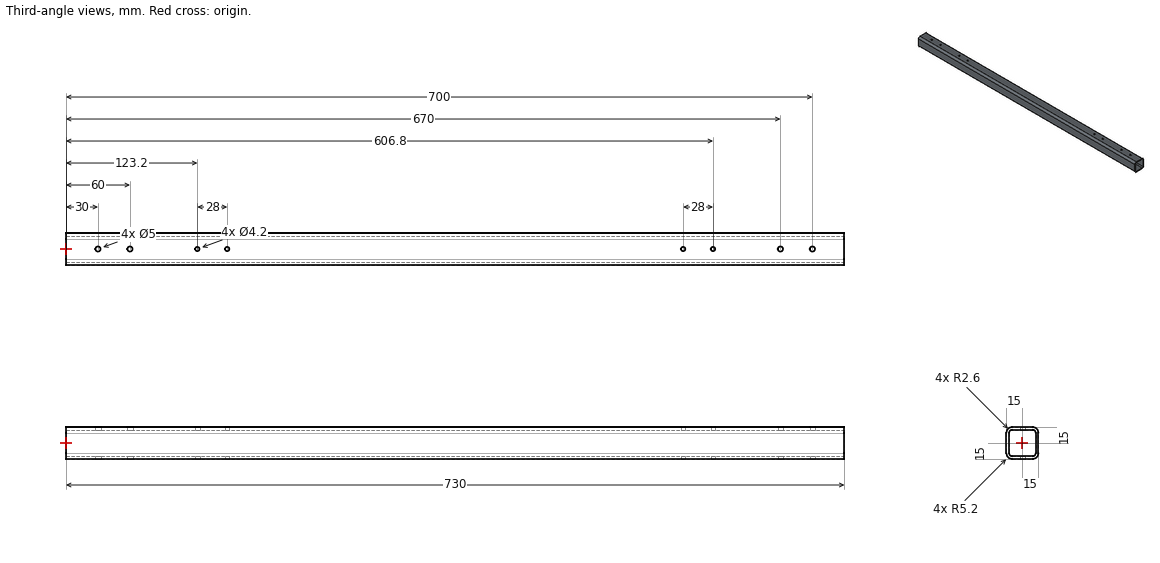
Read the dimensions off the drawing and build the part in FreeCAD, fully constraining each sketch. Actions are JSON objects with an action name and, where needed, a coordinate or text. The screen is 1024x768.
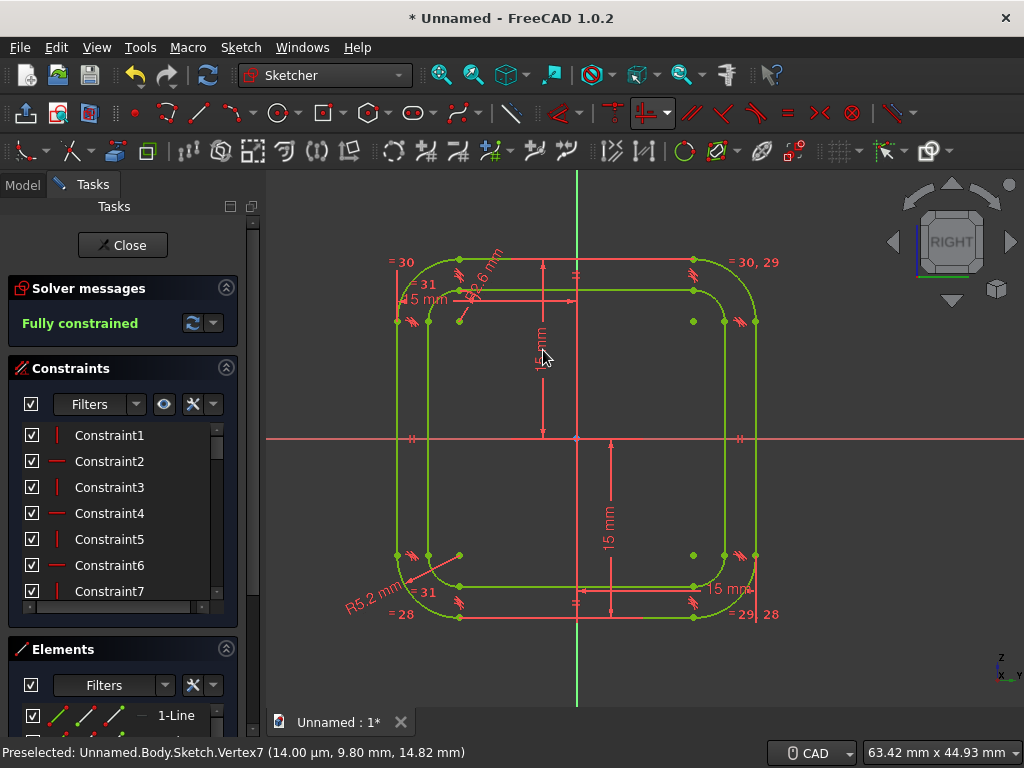
{"action": "left_click", "coordinate": [123, 245]}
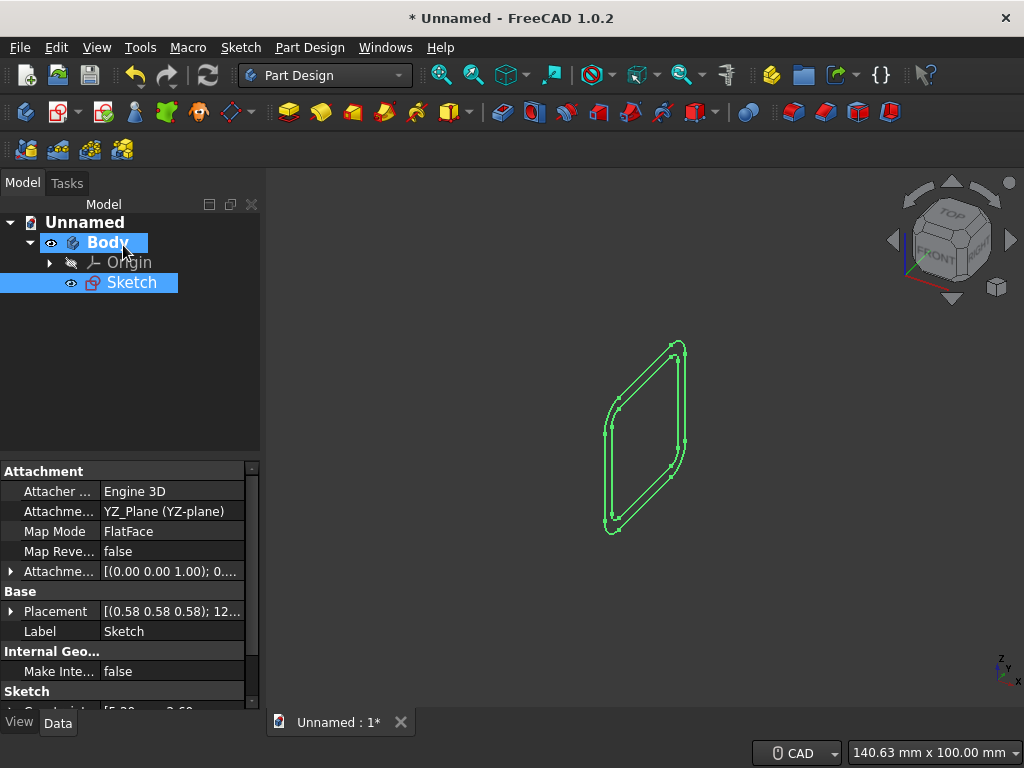
{"action": "left_click", "coordinate": [290, 112]}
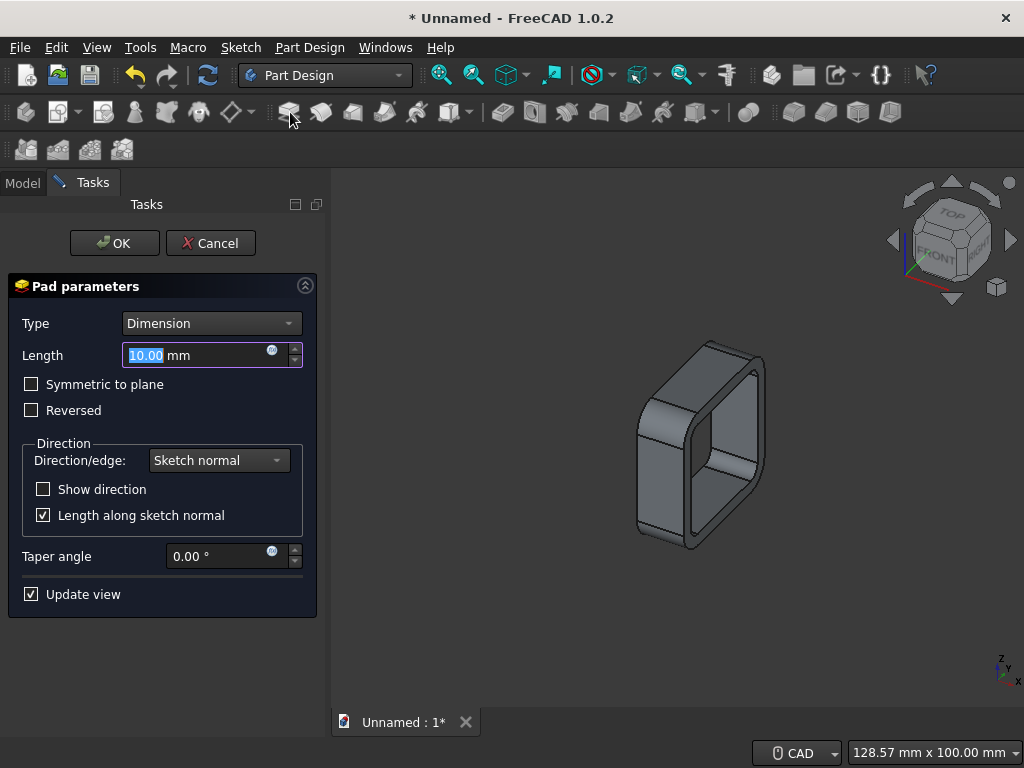
{"action": "type", "text": "730"}
{"action": "key", "text": "Tab"}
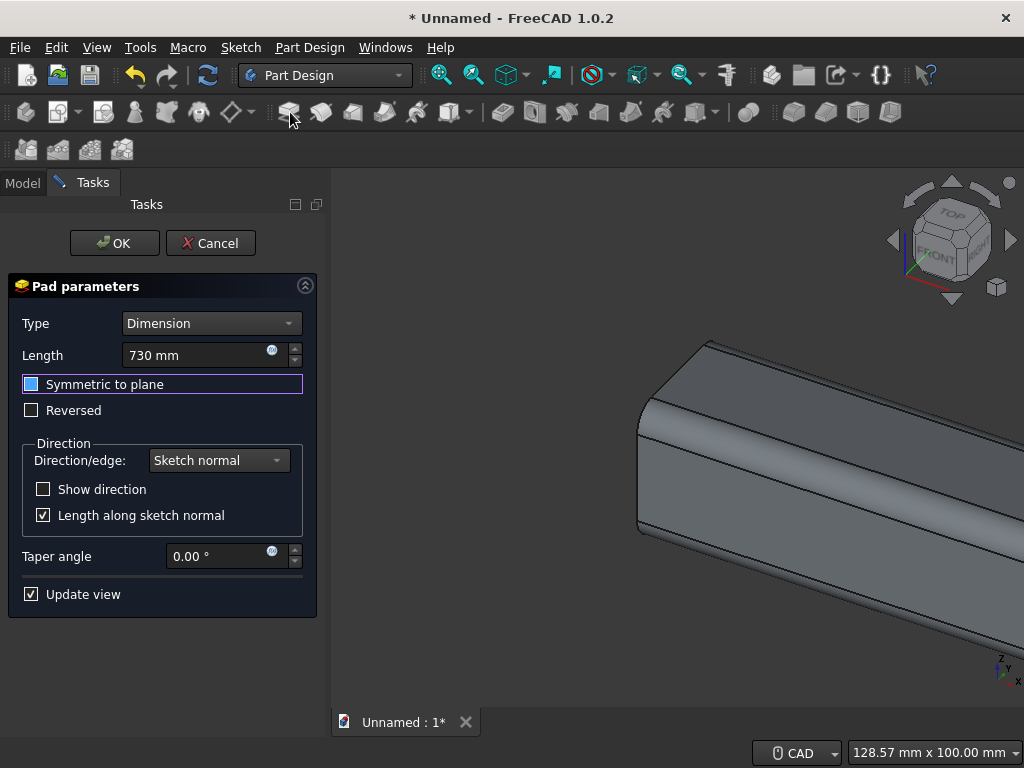
{"action": "left_click", "coordinate": [115, 243]}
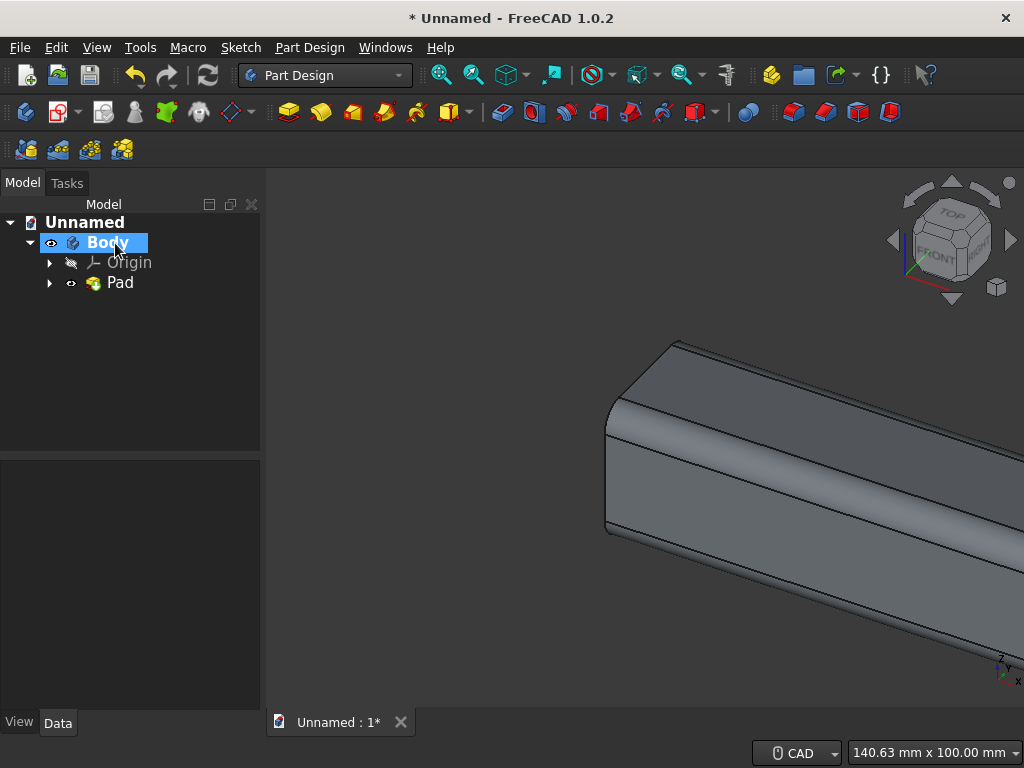
{"action": "left_click", "coordinate": [442, 76]}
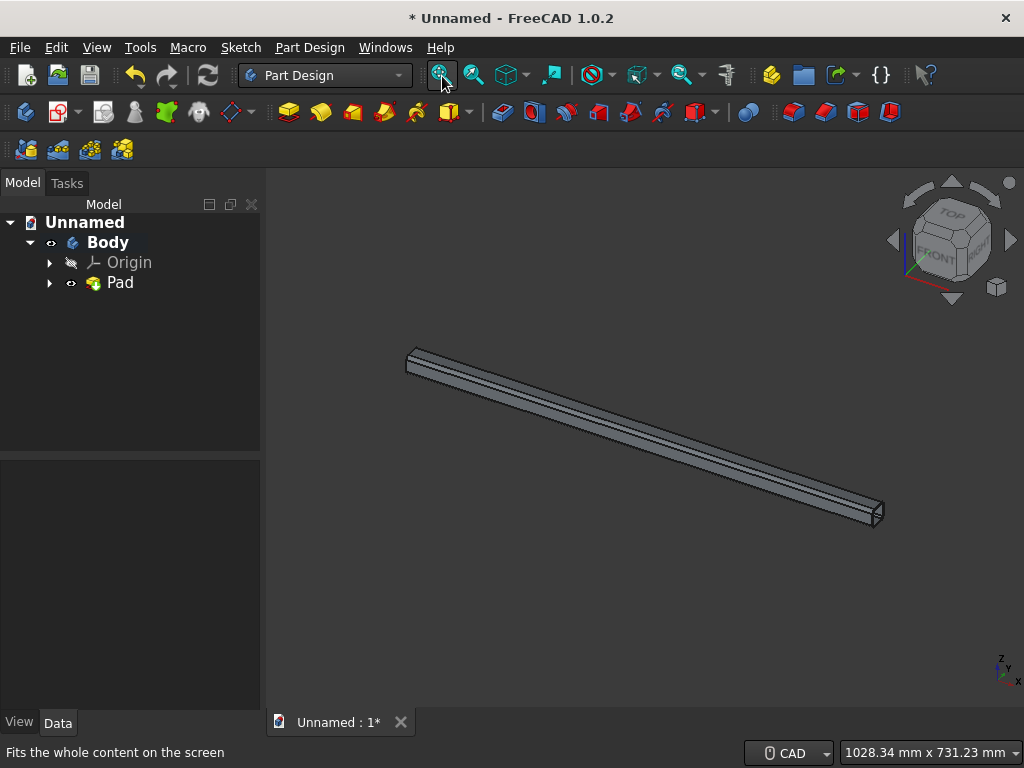
{"action": "key", "text": "0"}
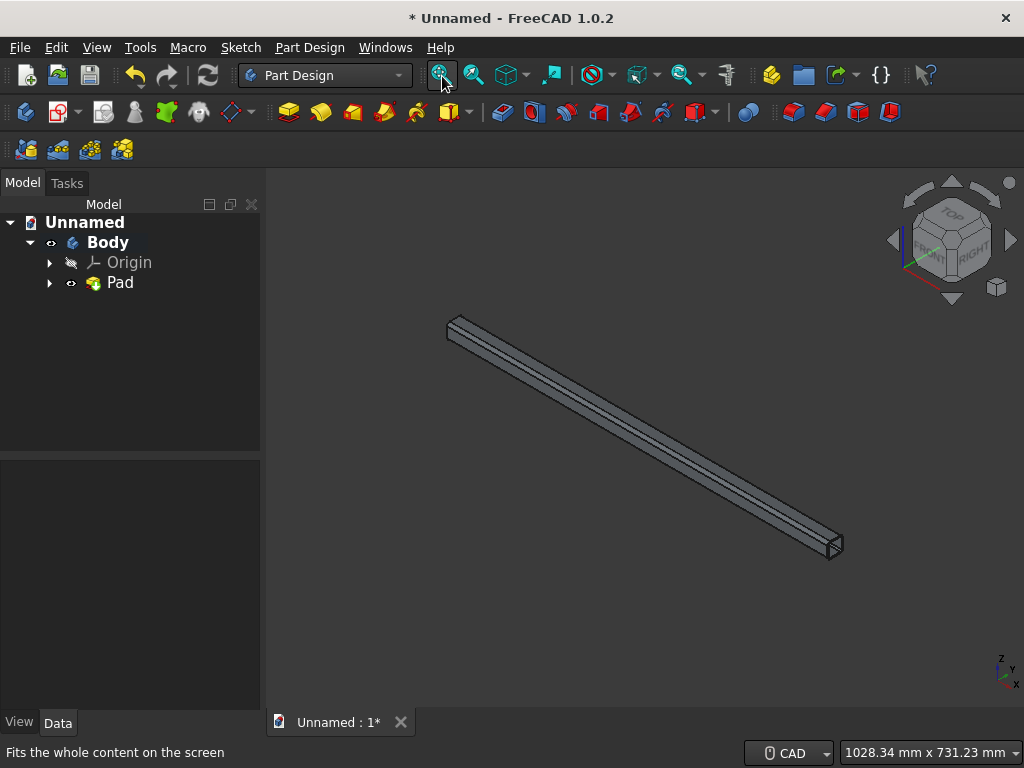
{"action": "key", "text": "2"}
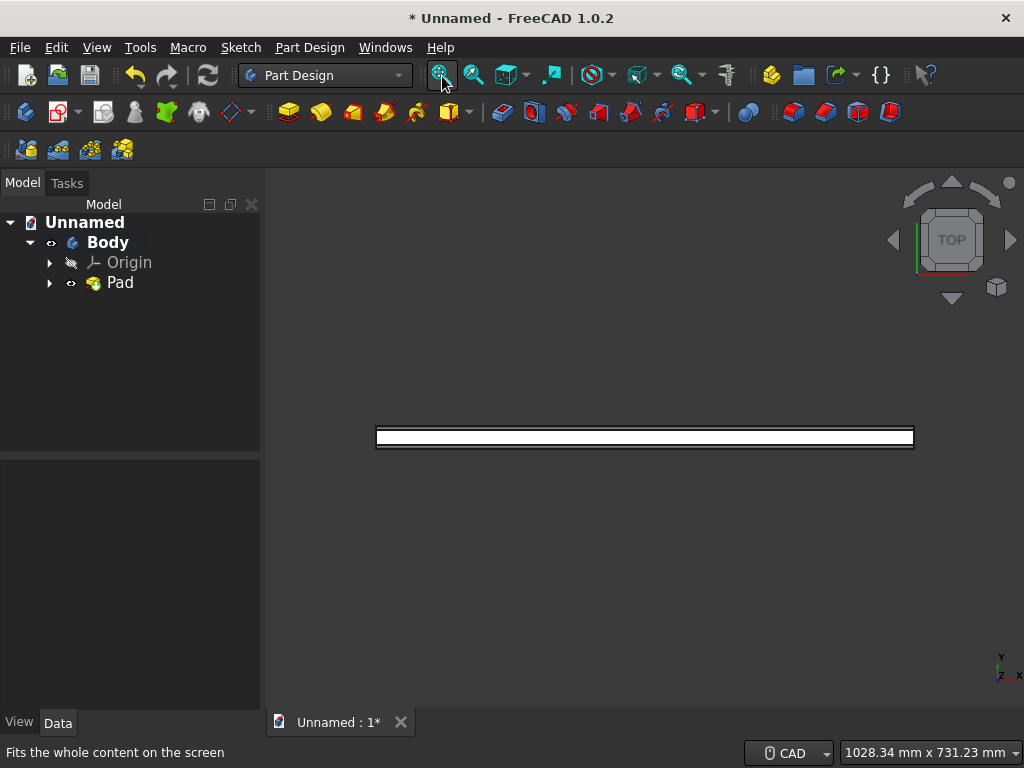
{"action": "key", "text": "4"}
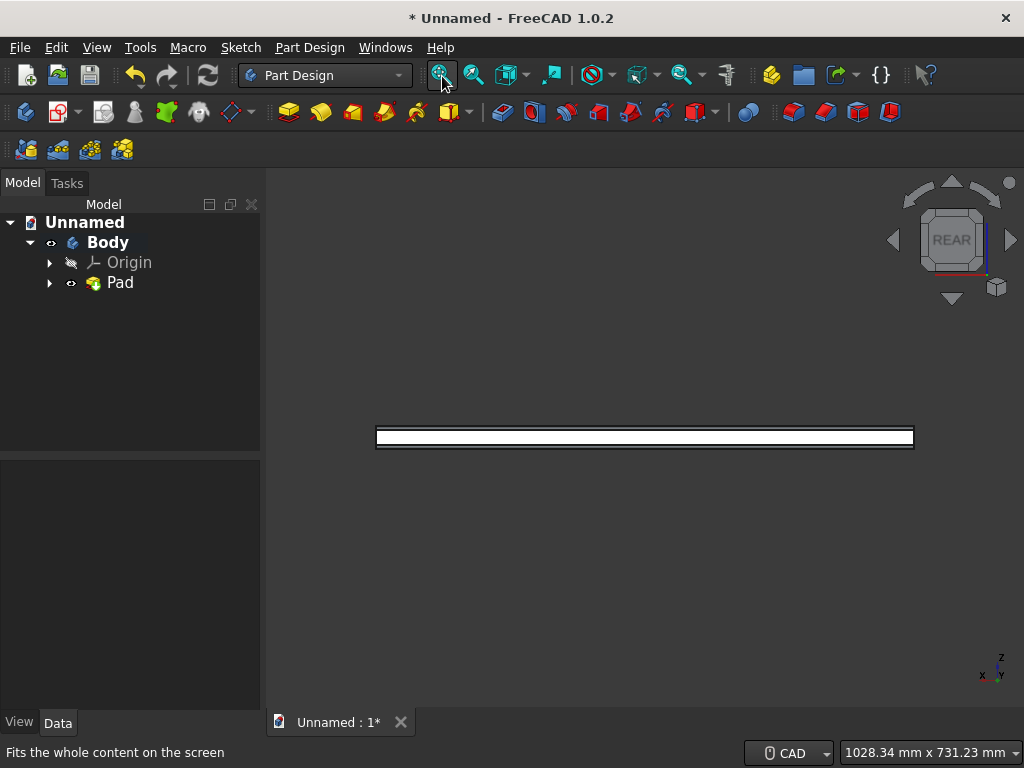
{"action": "left_click", "coordinate": [50, 263]}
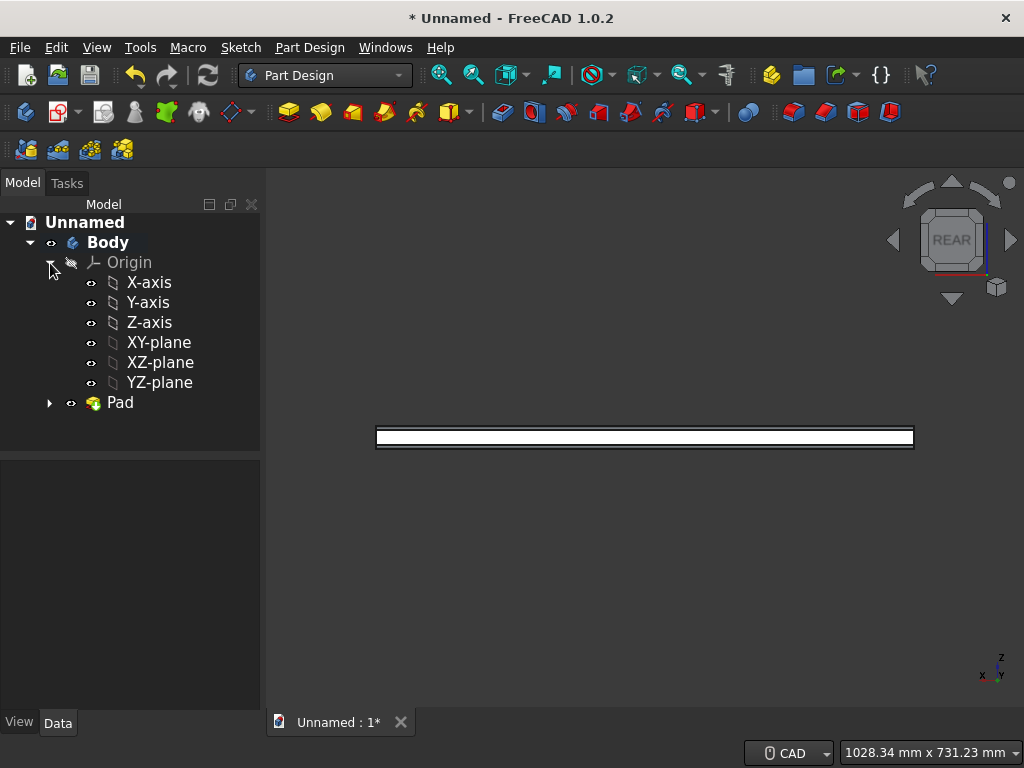
{"action": "left_click", "coordinate": [136, 343]}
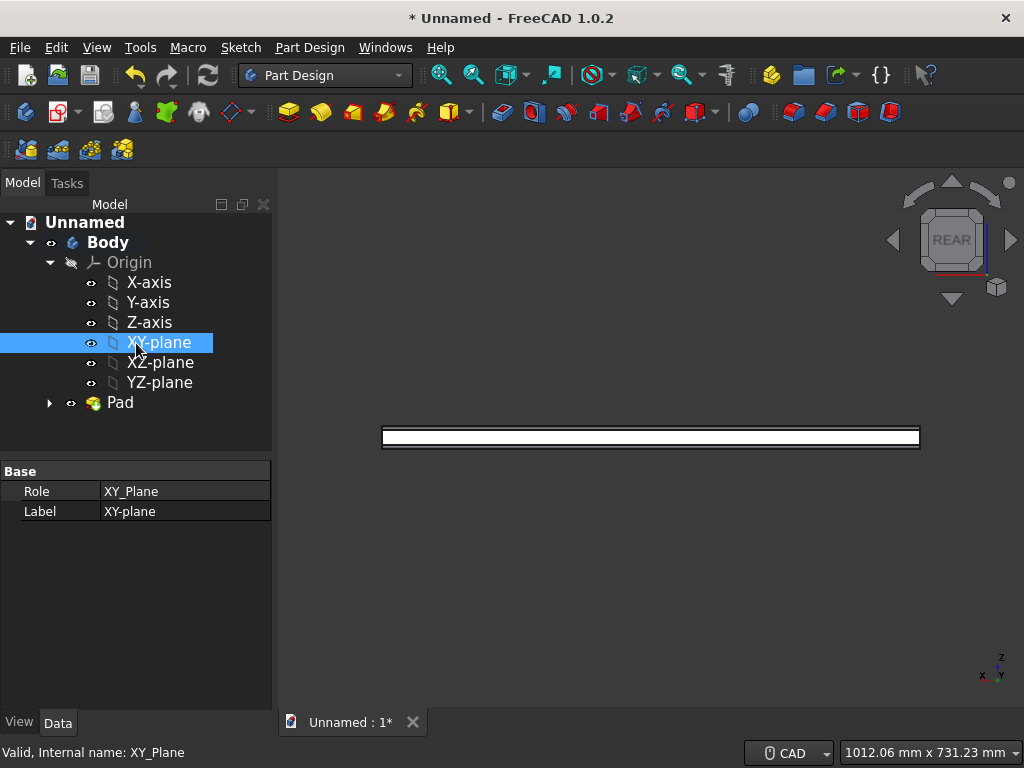
{"action": "left_click", "coordinate": [232, 112]}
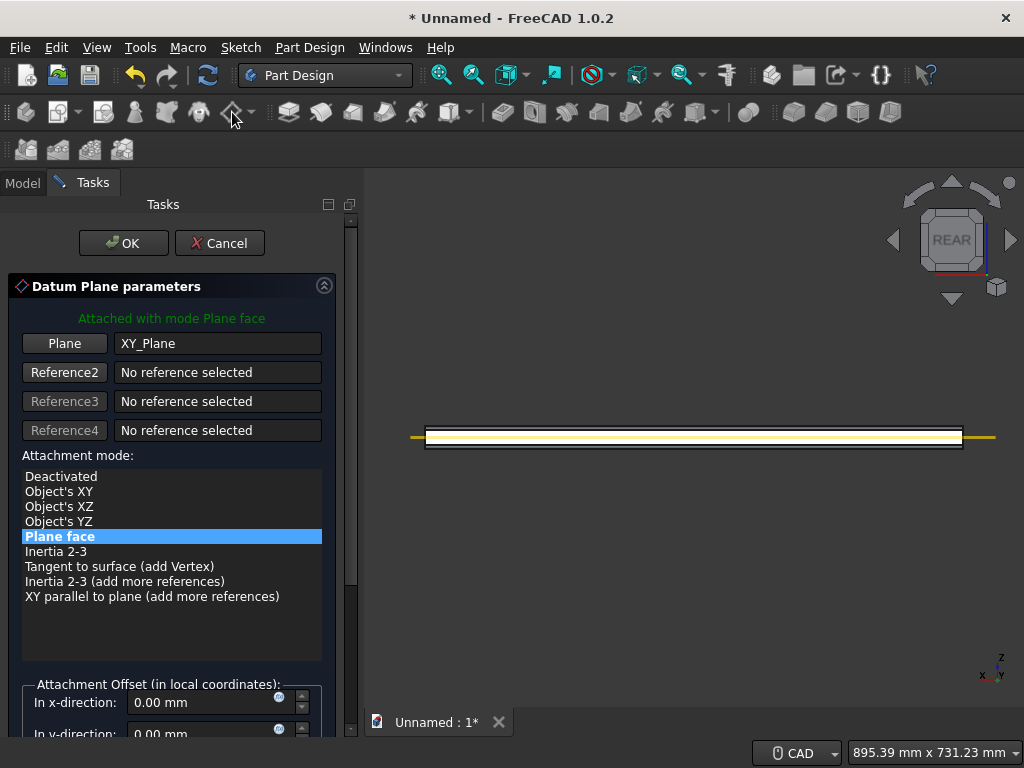
{"action": "scroll", "coordinate": [351, 475], "scroll_direction": "down", "scroll_amount": 2}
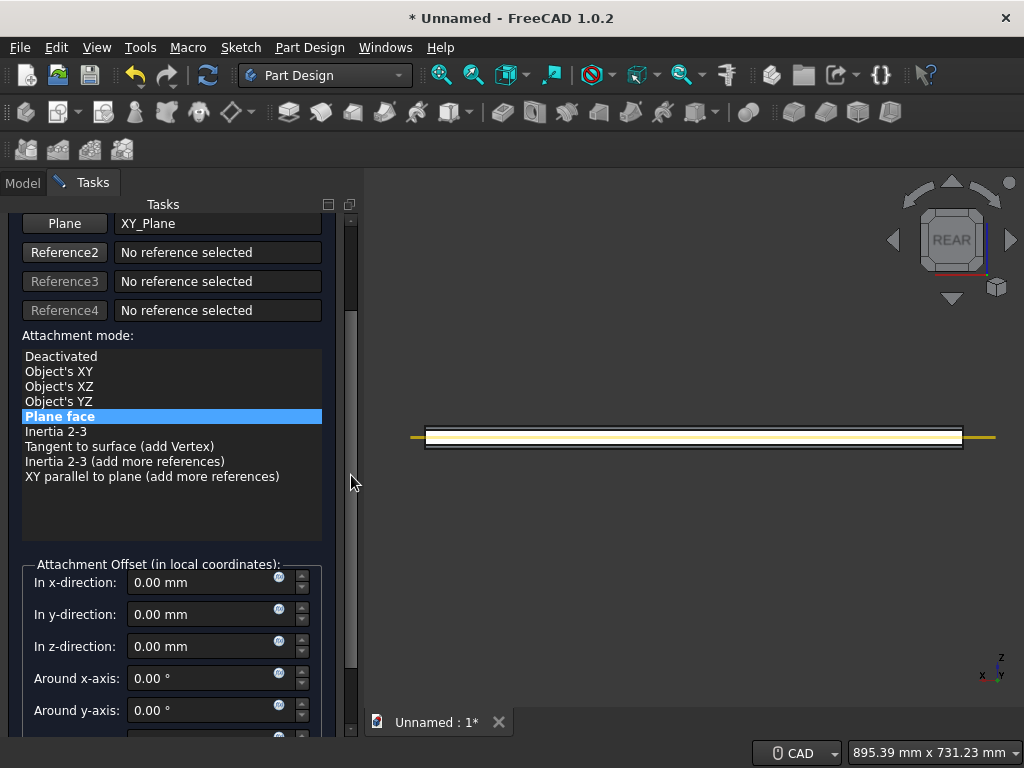
{"action": "triple_click", "coordinate": [210, 646]}